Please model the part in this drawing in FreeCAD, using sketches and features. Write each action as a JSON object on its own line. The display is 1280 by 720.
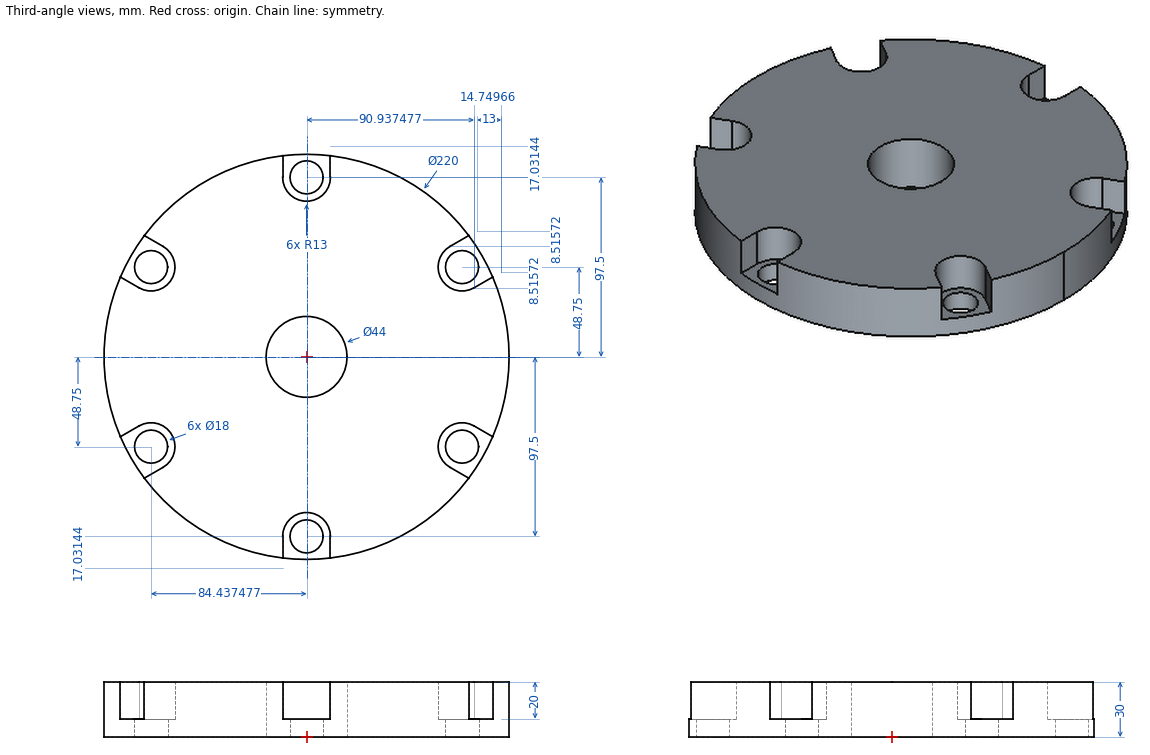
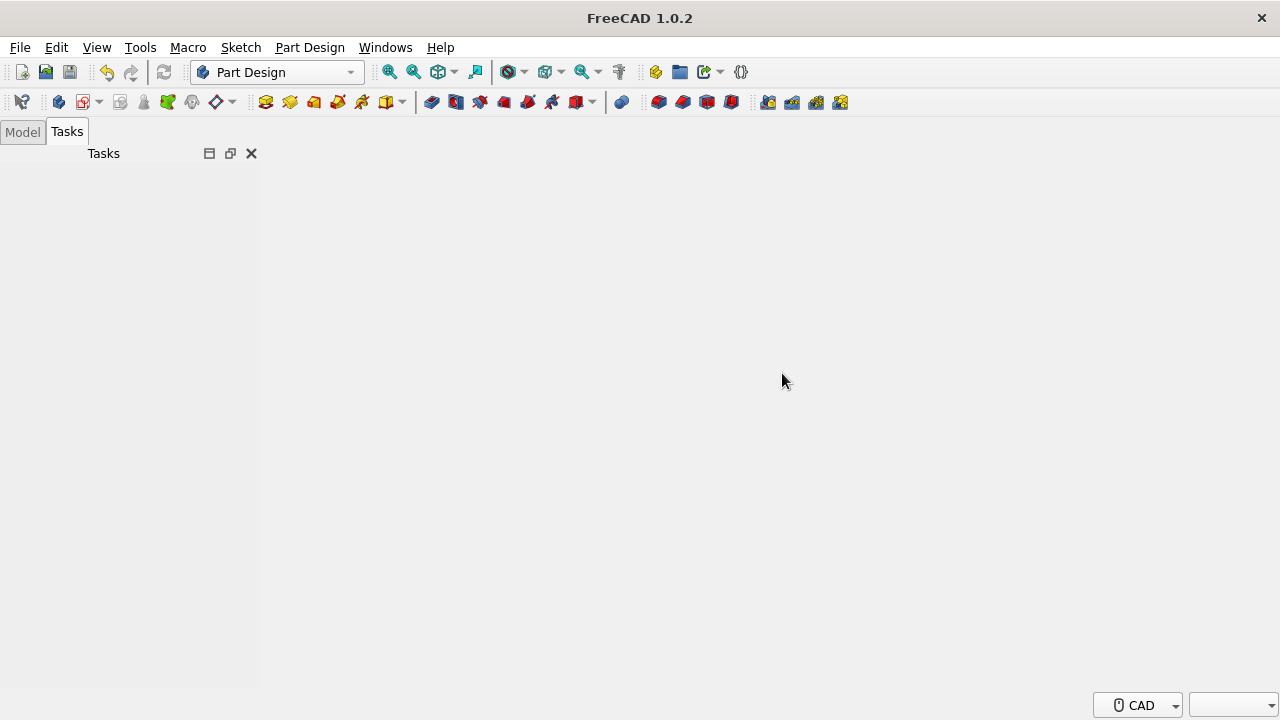
{"action": "left_click", "coordinate": [22, 72]}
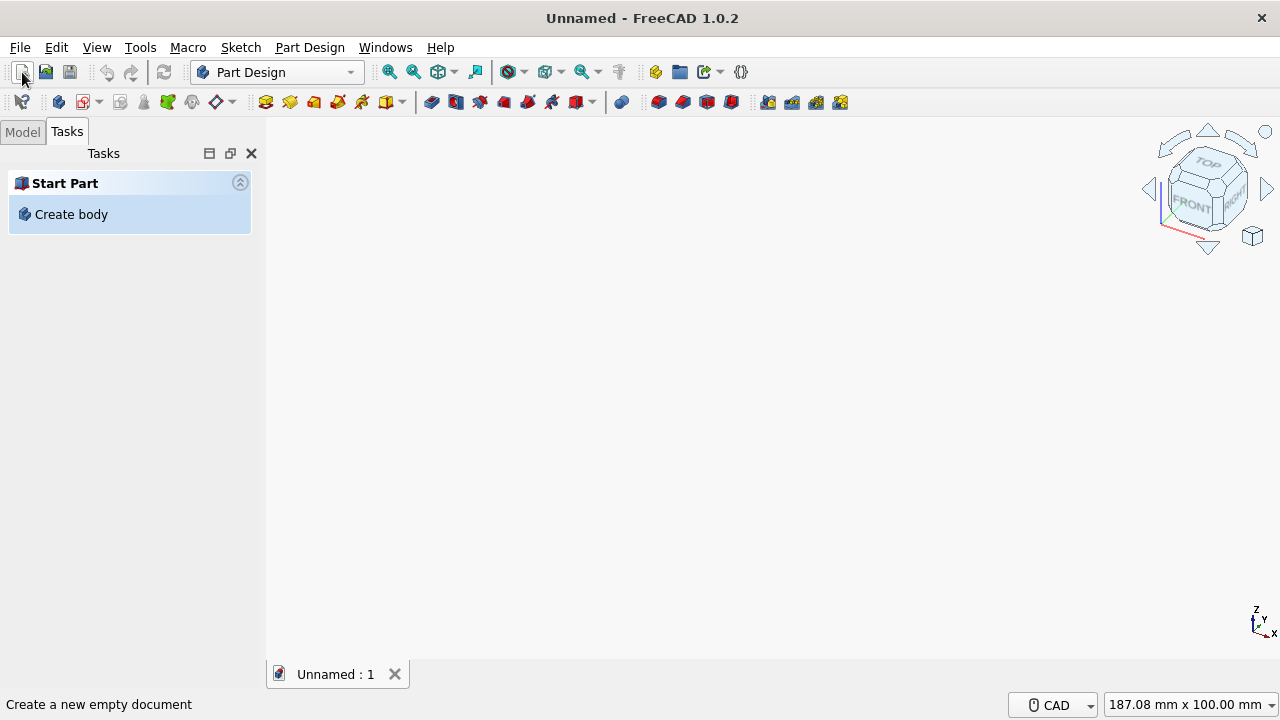
{"action": "left_click", "coordinate": [84, 102]}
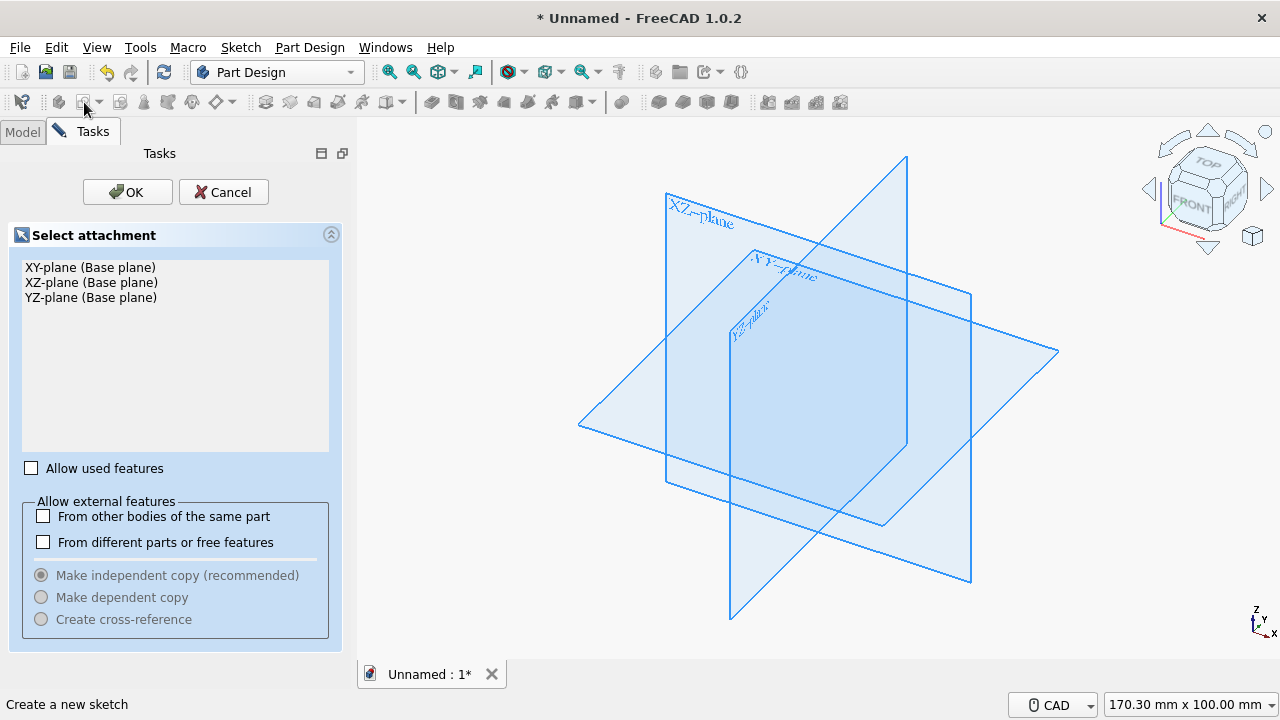
{"action": "left_click", "coordinate": [82, 268]}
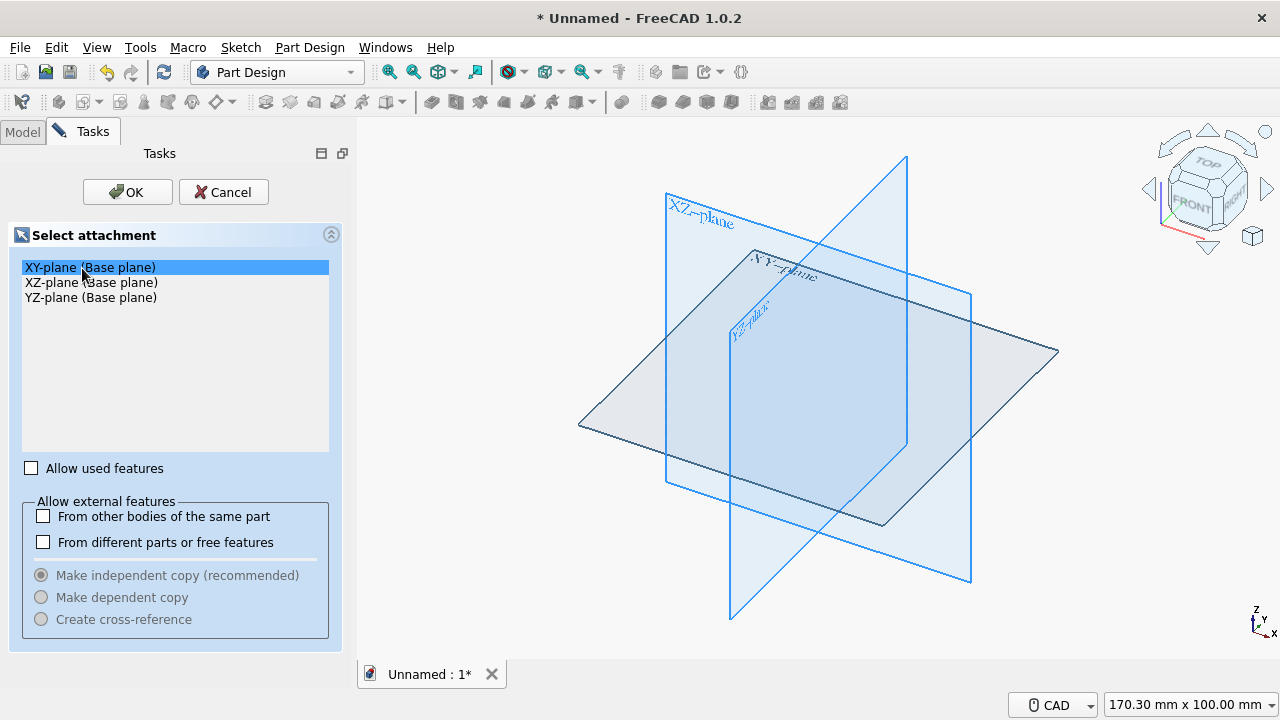
{"action": "left_click", "coordinate": [128, 192]}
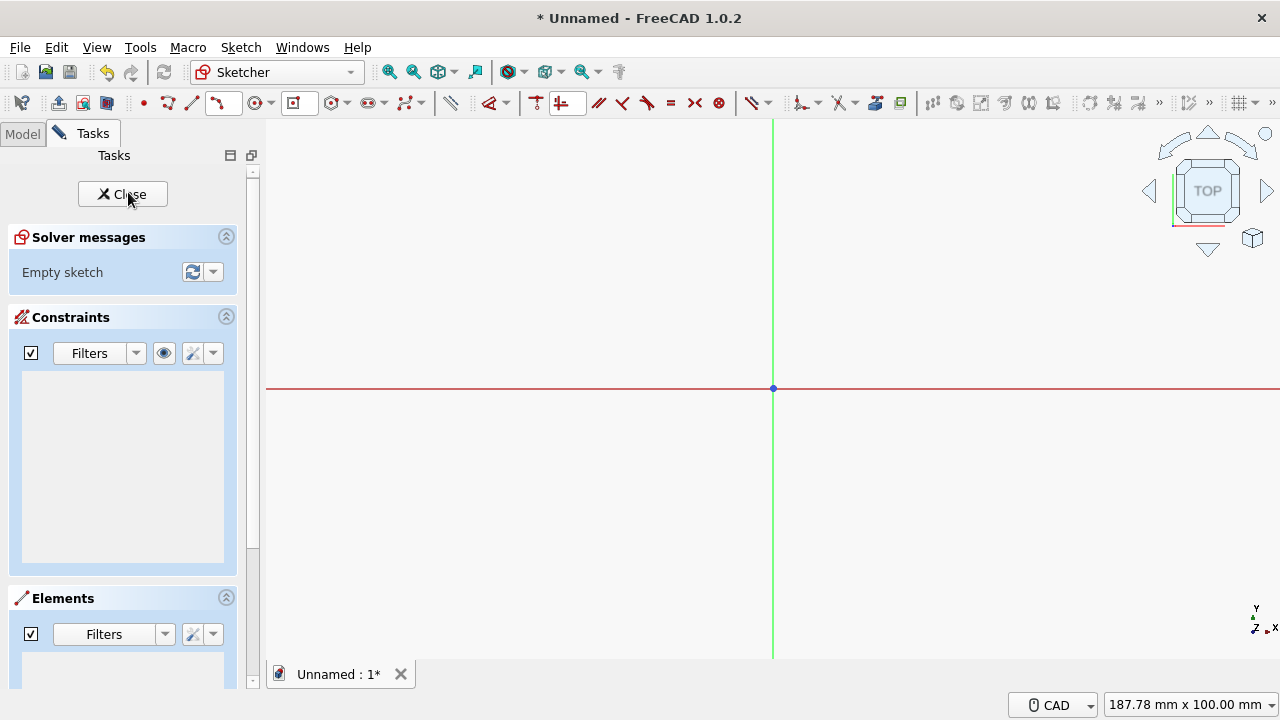
{"action": "scroll", "coordinate": [675, 389], "scroll_direction": "down", "scroll_amount": 6}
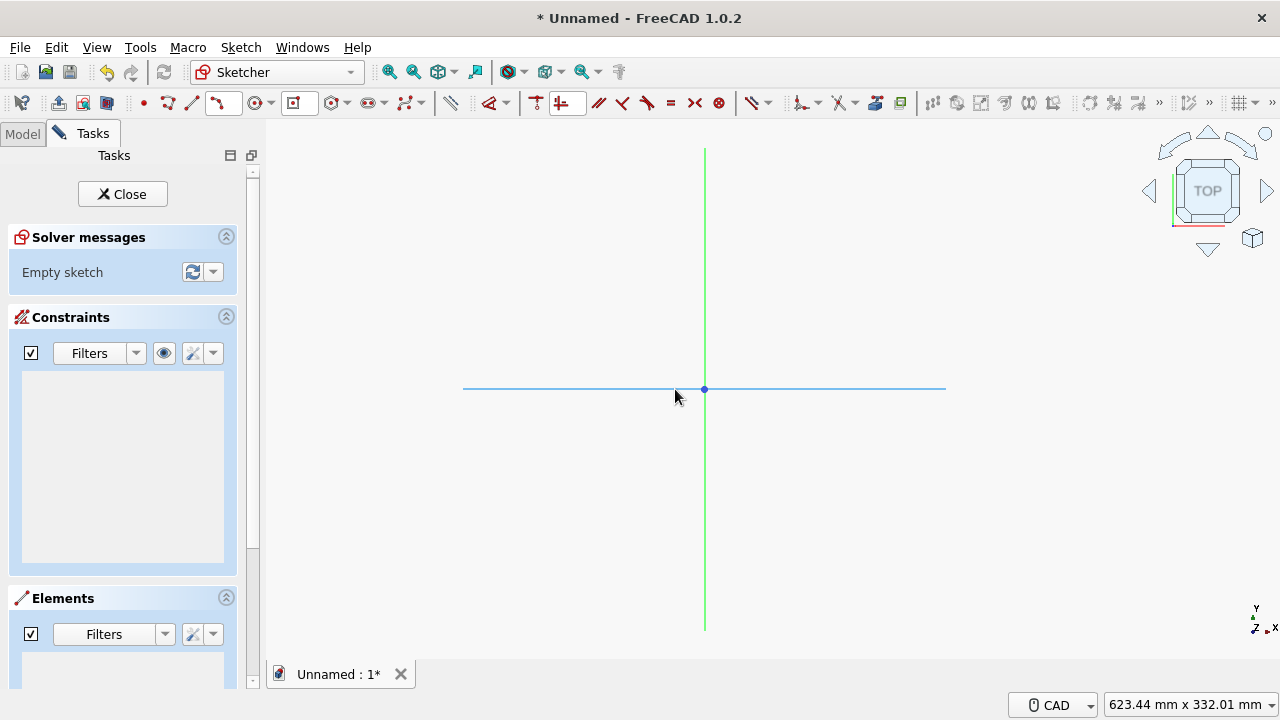
{"action": "left_click", "coordinate": [256, 104]}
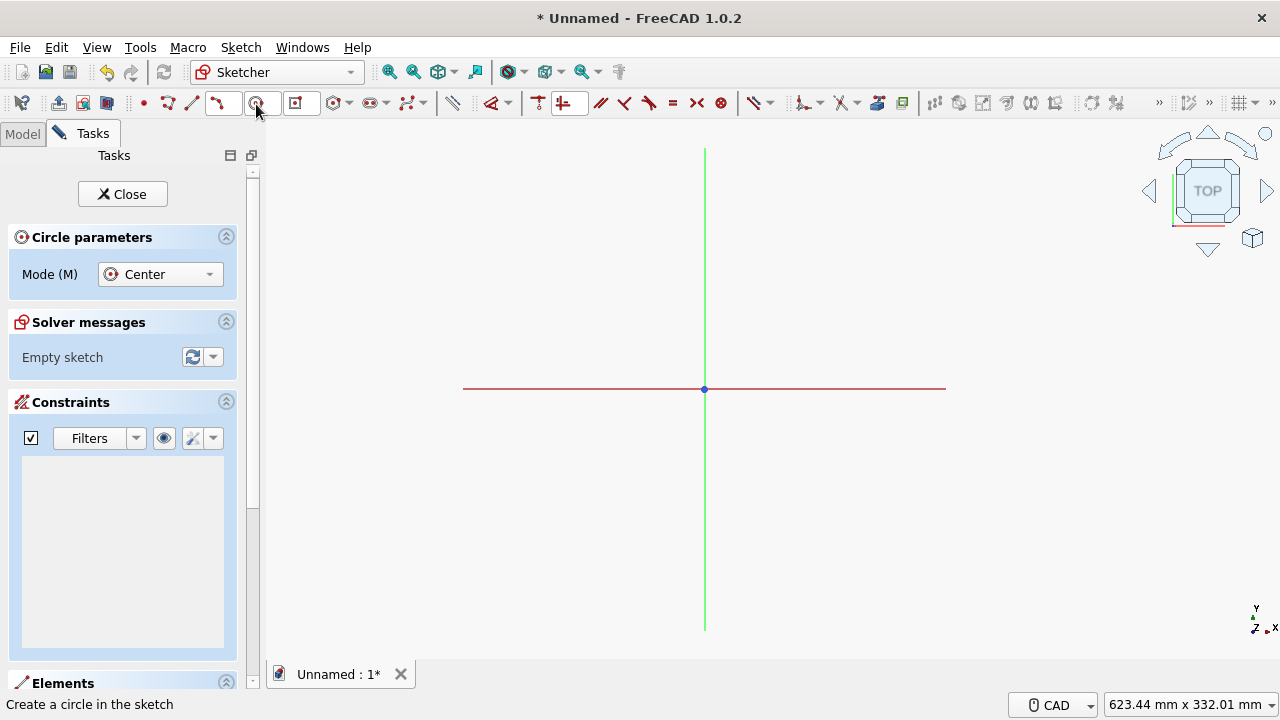
{"action": "left_click", "coordinate": [705, 389]}
{"action": "mouse_move", "coordinate": [831, 263]}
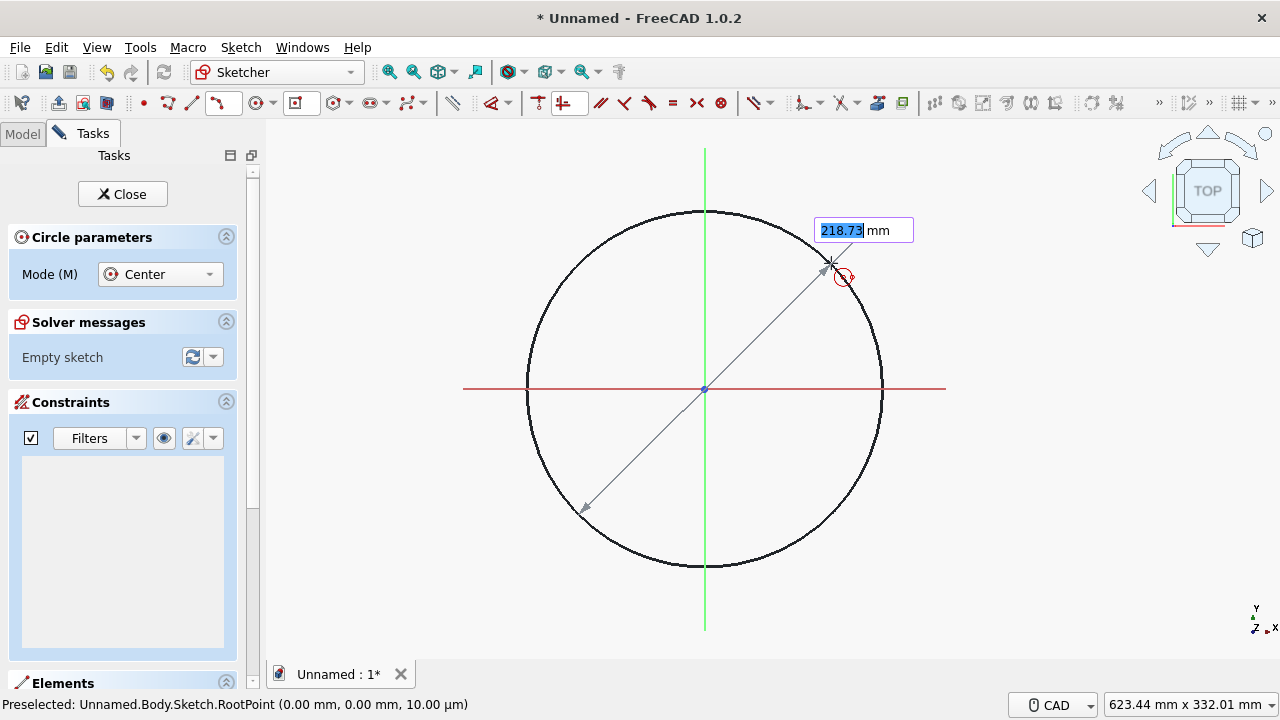
{"action": "type", "text": "220"}
{"action": "key", "text": "Return"}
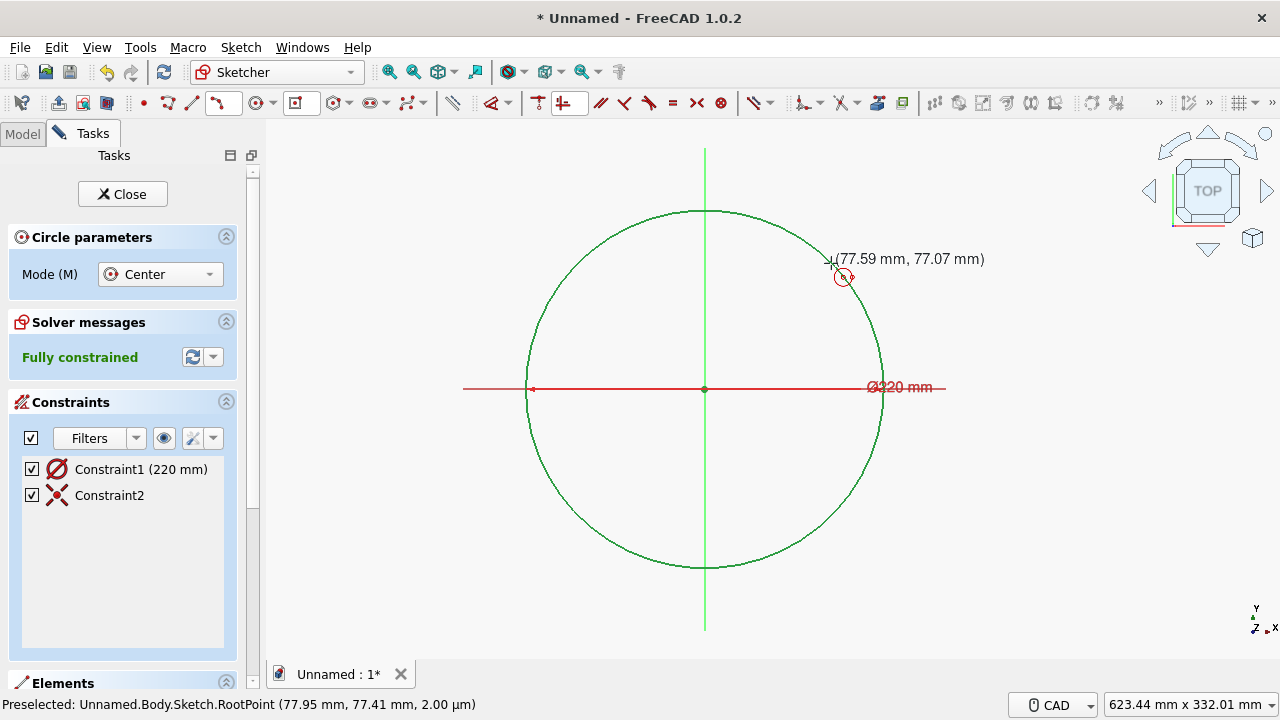
{"action": "scroll", "coordinate": [567, 469], "scroll_direction": "up", "scroll_amount": 3}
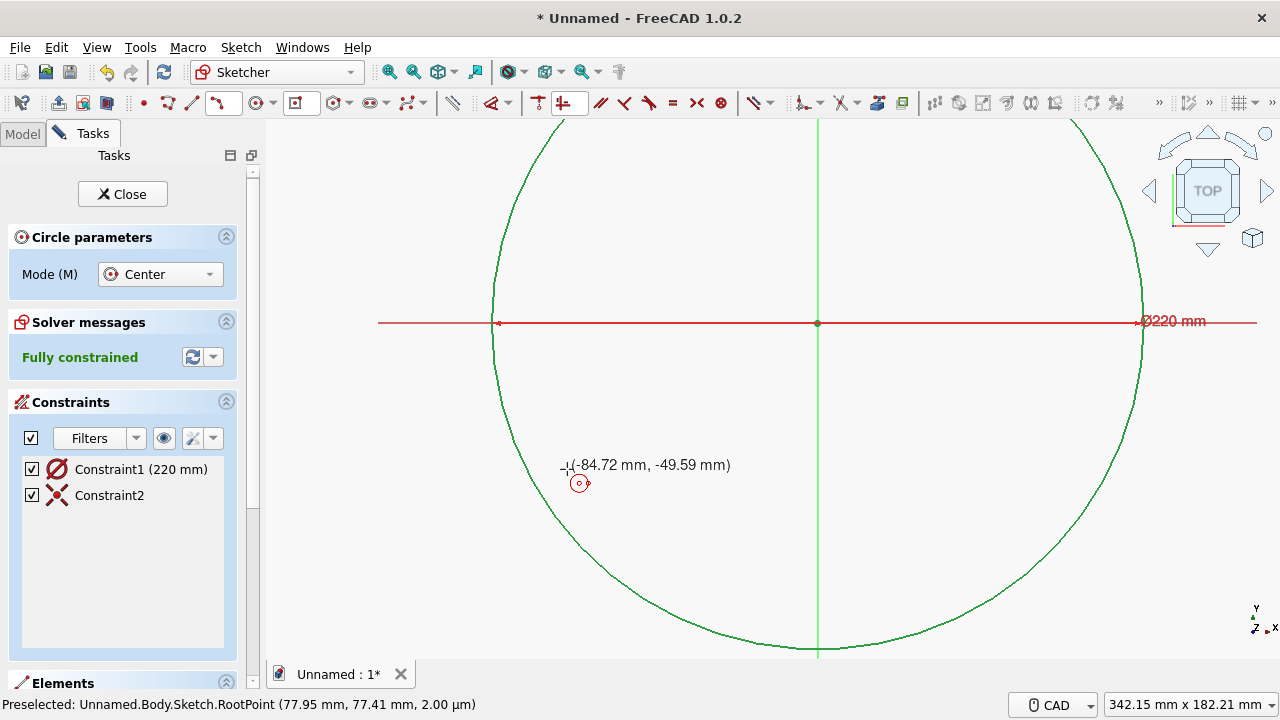
{"action": "left_click", "coordinate": [568, 468]}
{"action": "mouse_move", "coordinate": [586, 449]}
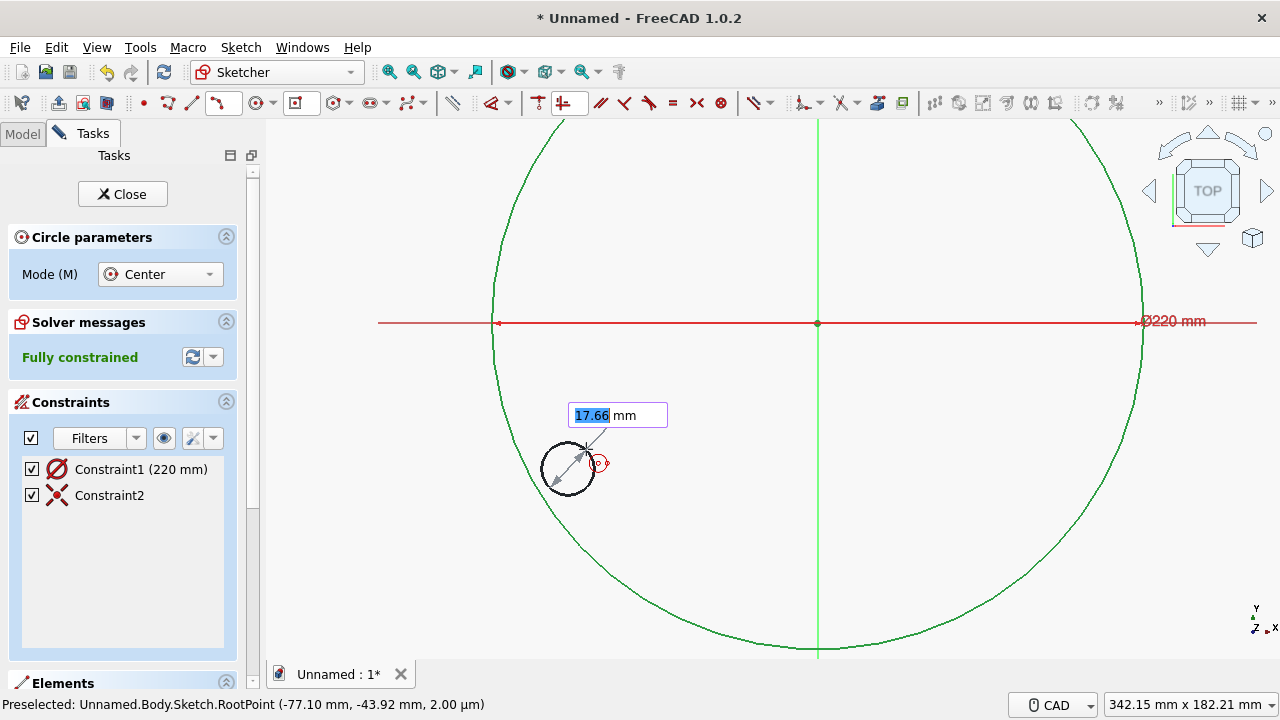
{"action": "type", "text": "18"}
{"action": "key", "text": "Return"}